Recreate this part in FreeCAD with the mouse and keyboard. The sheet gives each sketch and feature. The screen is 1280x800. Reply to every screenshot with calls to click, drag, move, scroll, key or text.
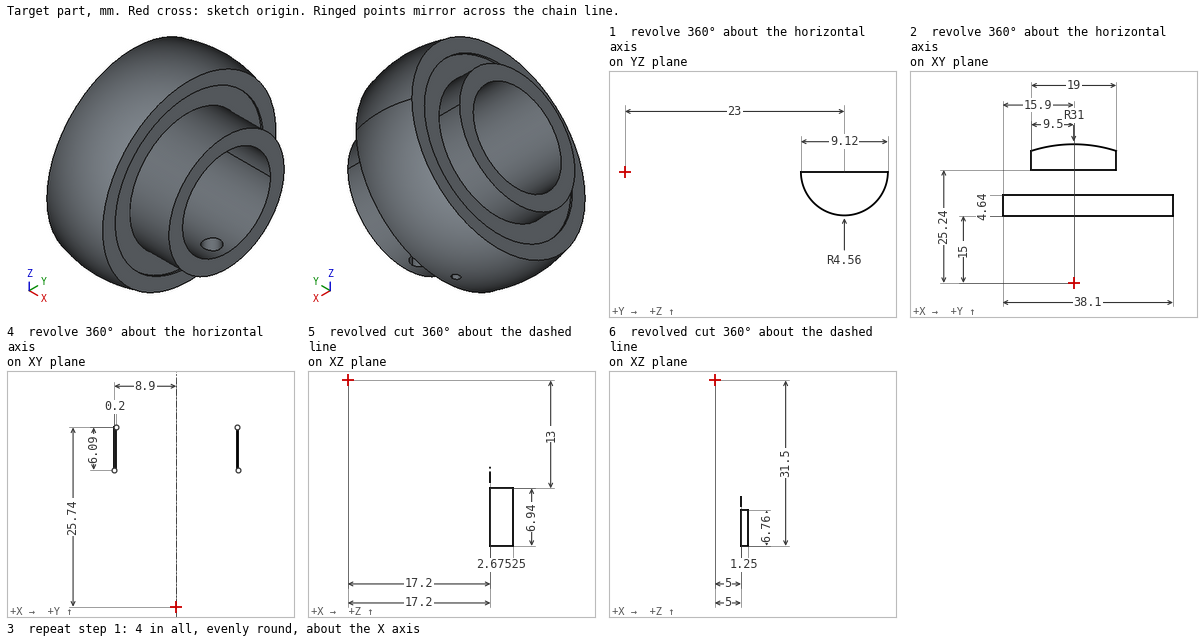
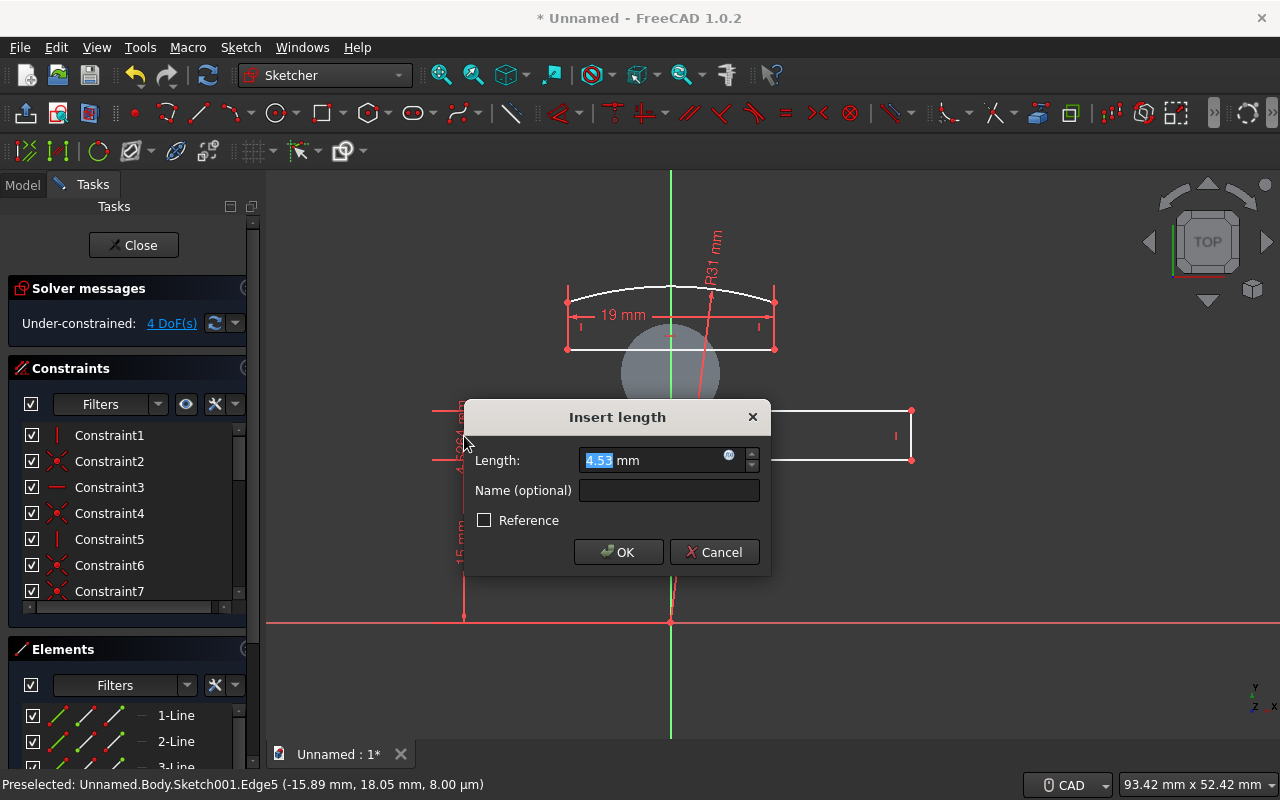
text(4.64)
key(Return)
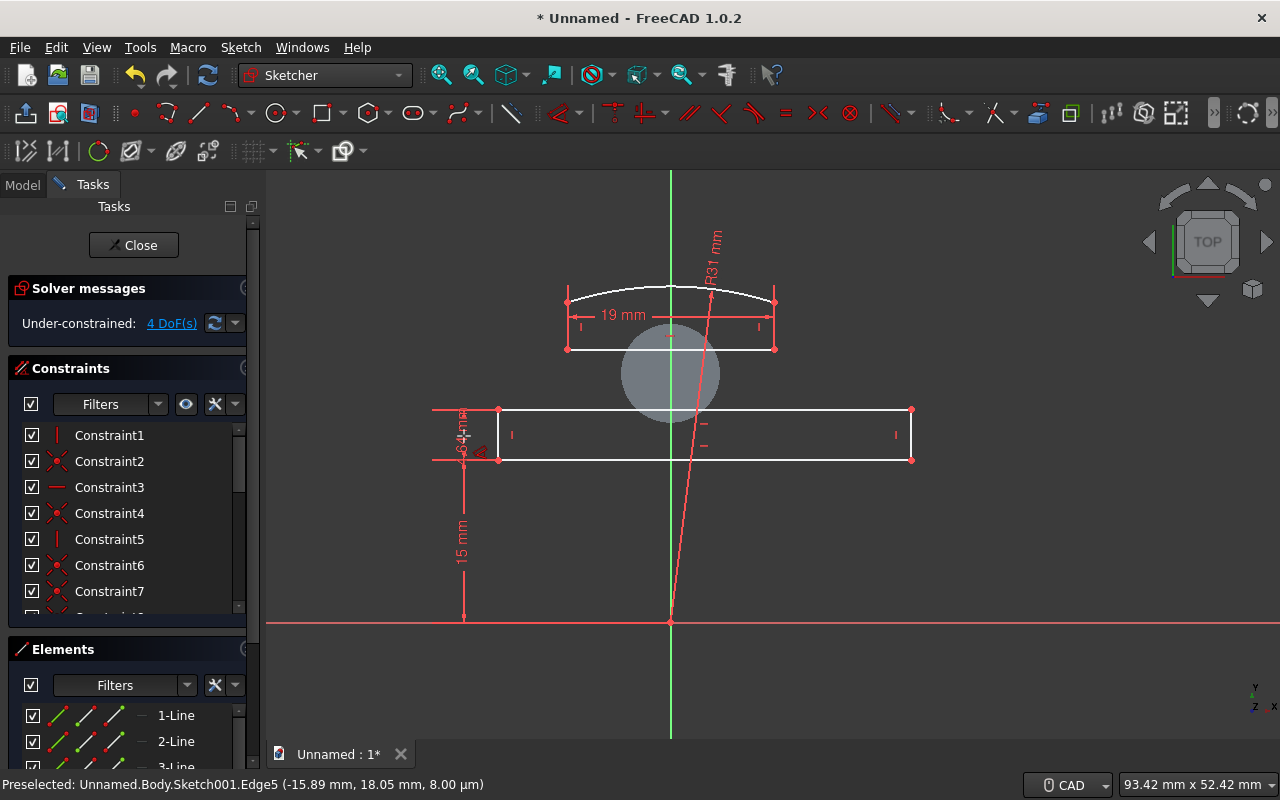
click(622, 460)
click(705, 494)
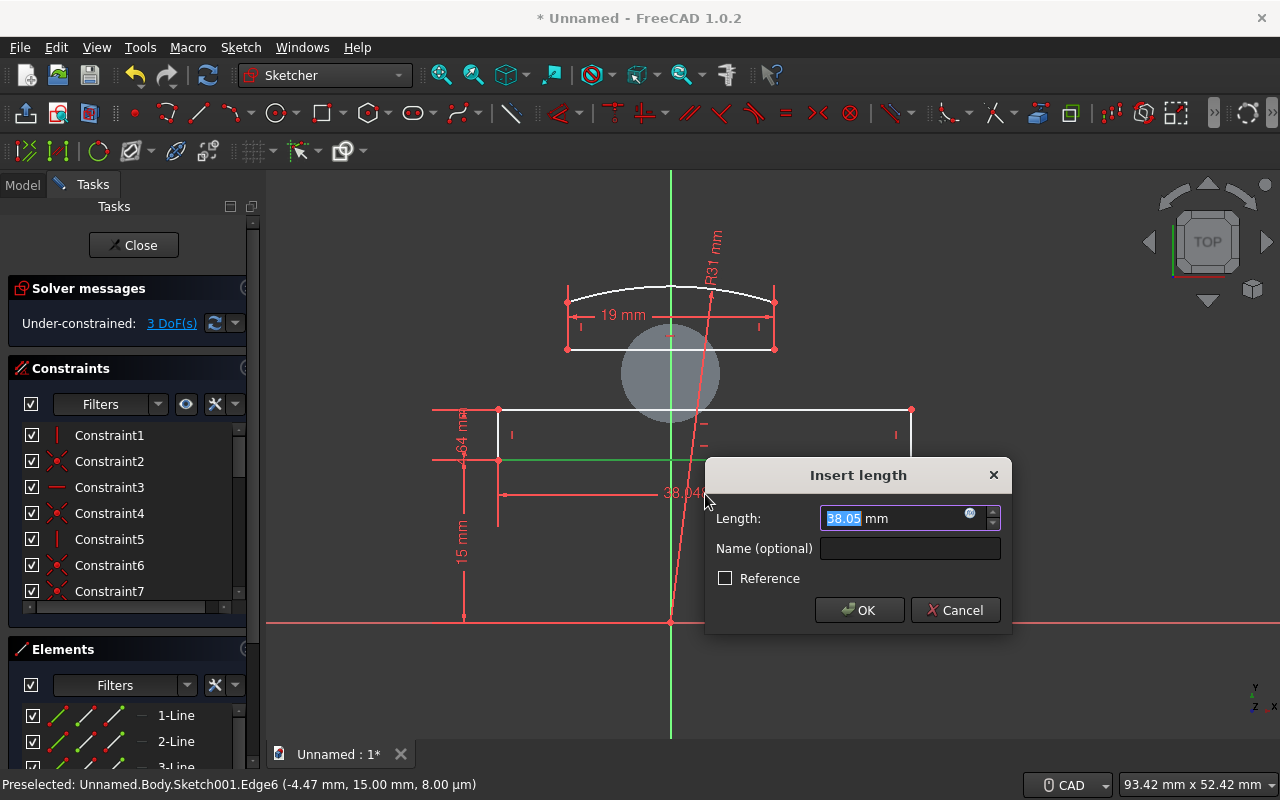
text(38.1)
key(Return)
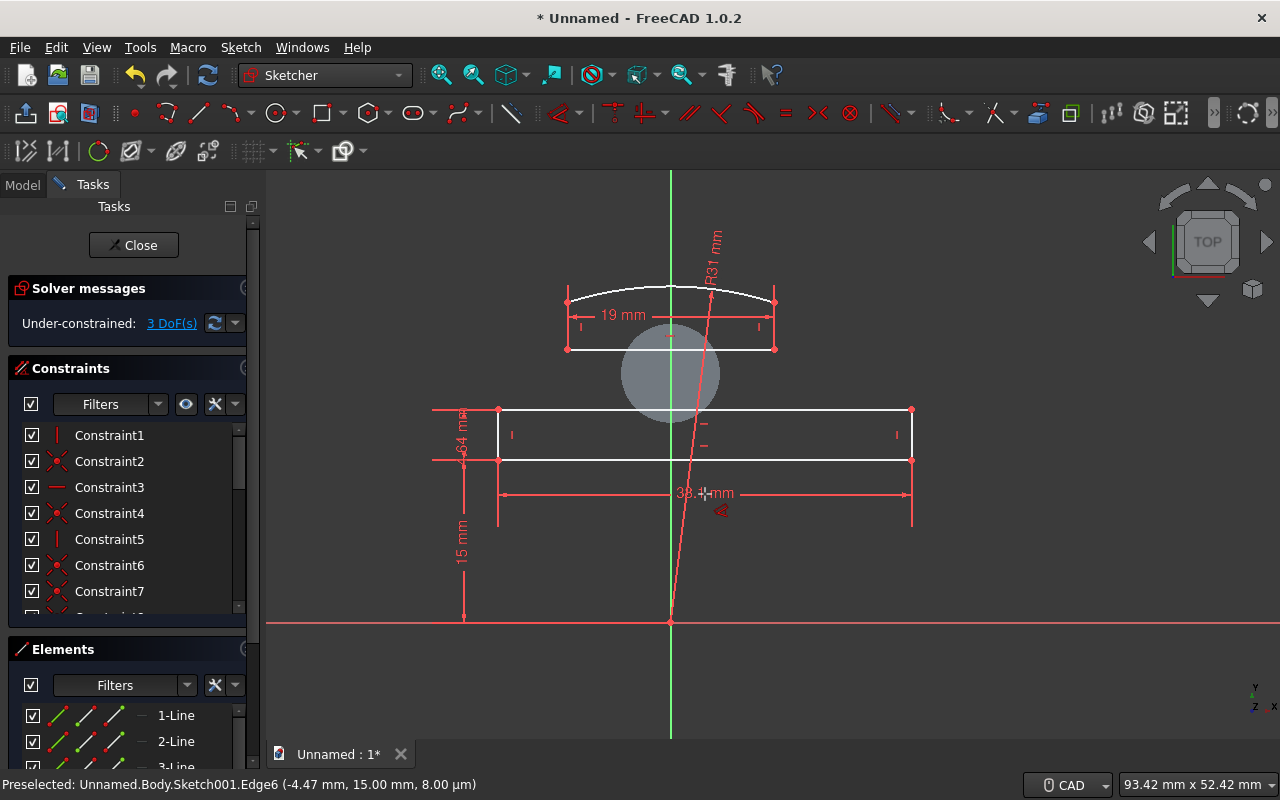
click(568, 303)
click(619, 657)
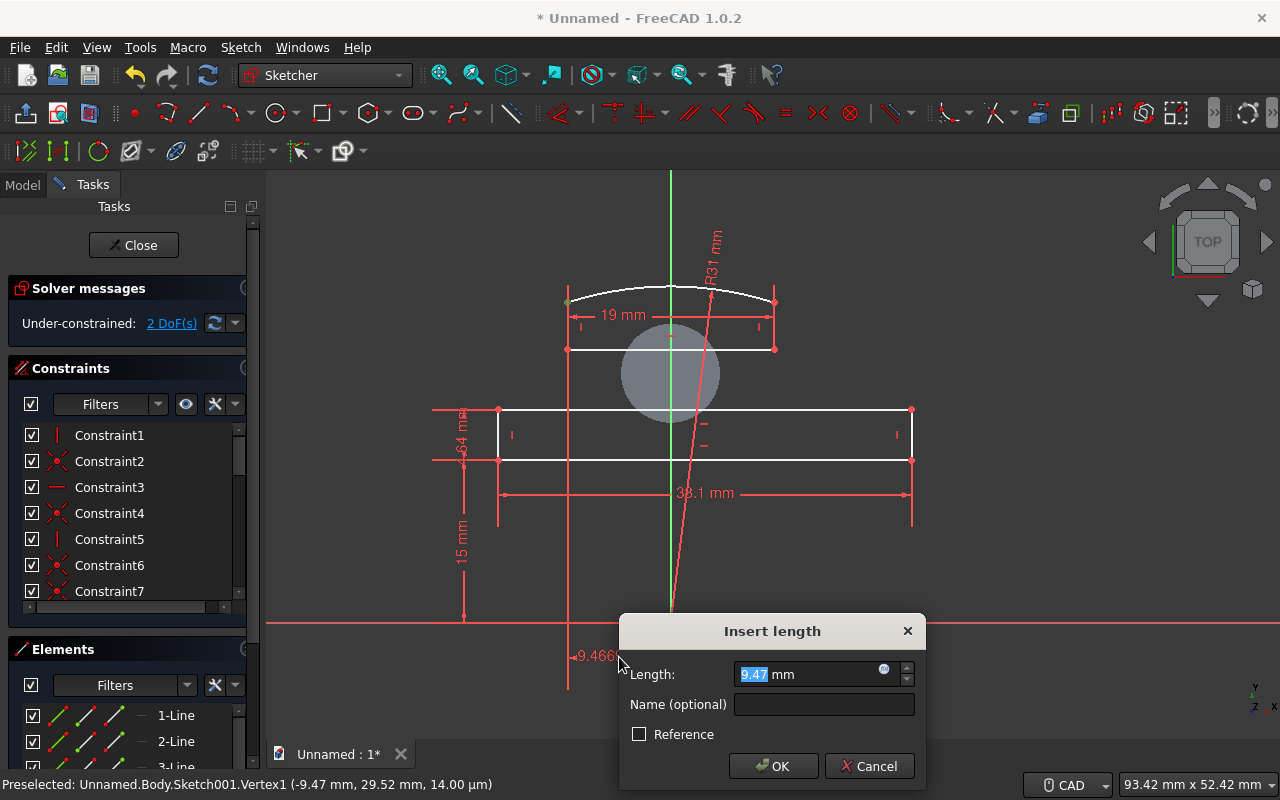
text(9.5)
key(Return)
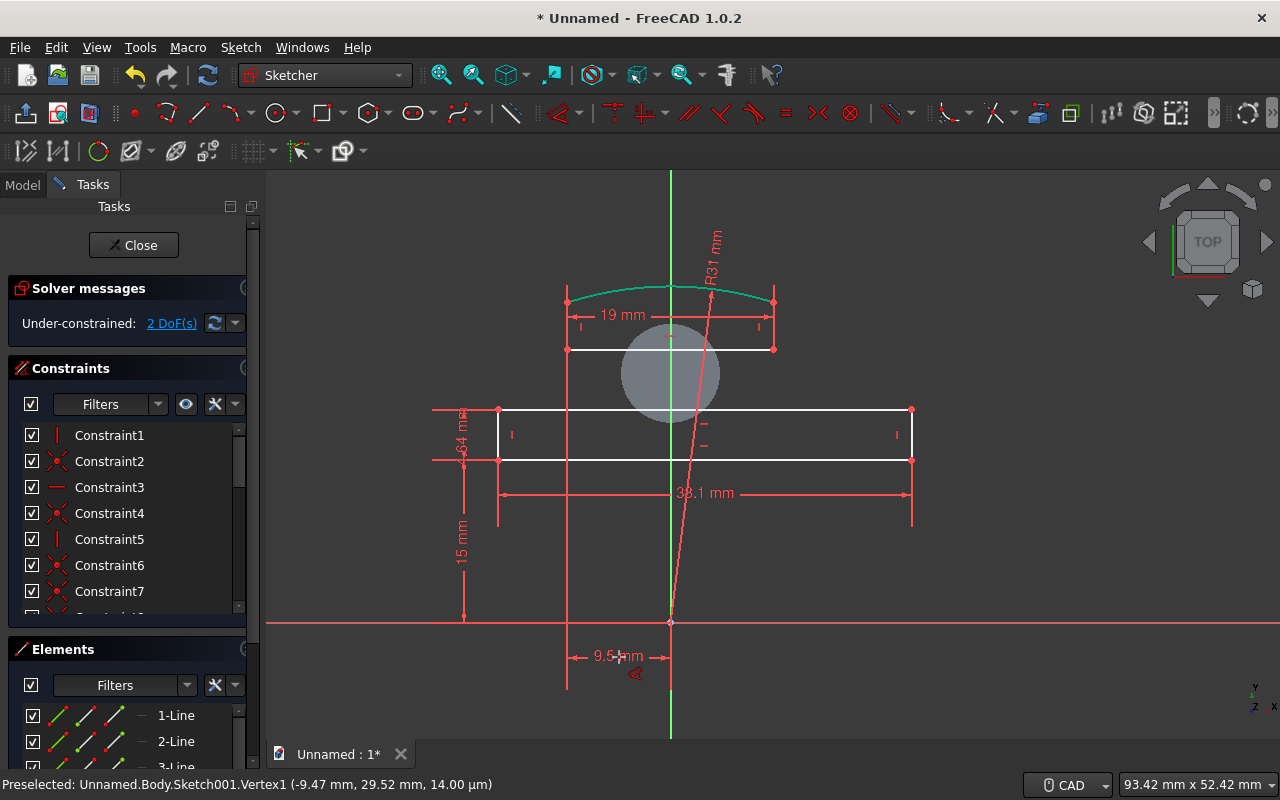
click(498, 410)
click(545, 657)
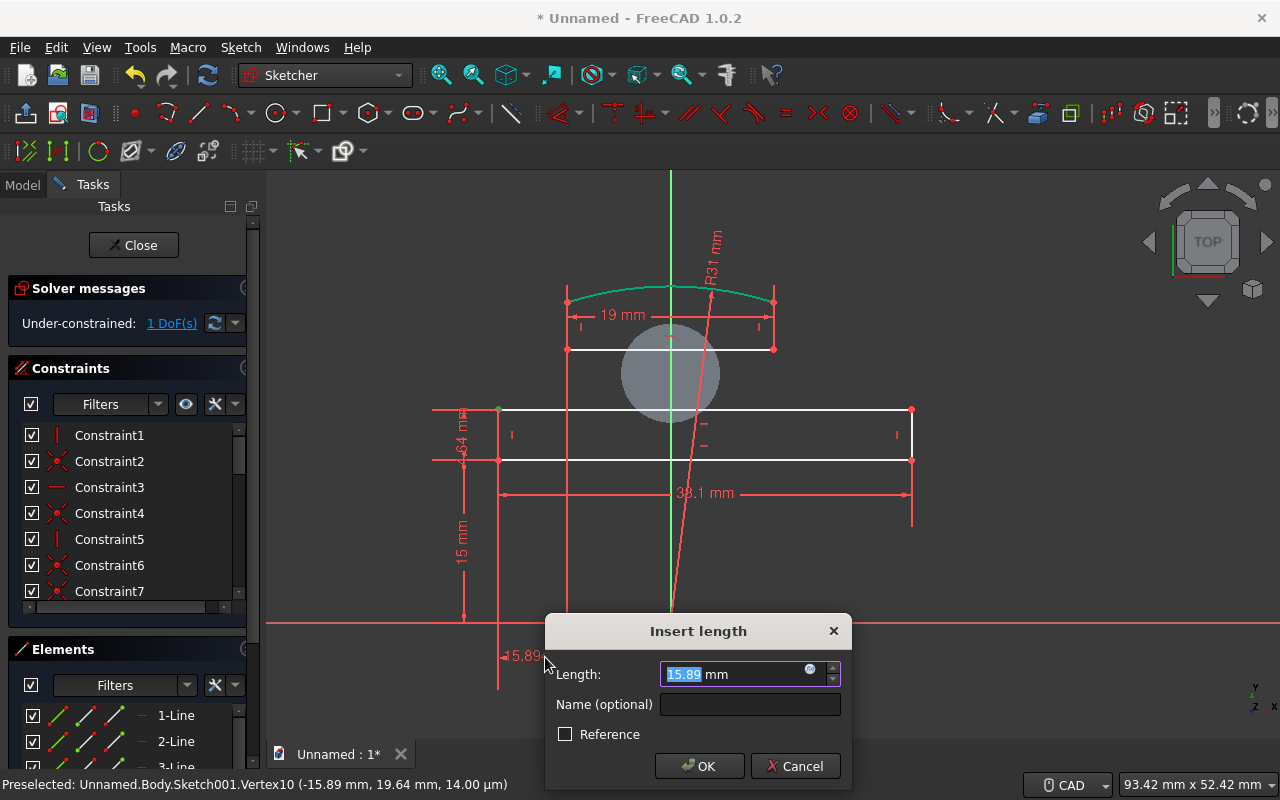
text(15.9)
key(Return)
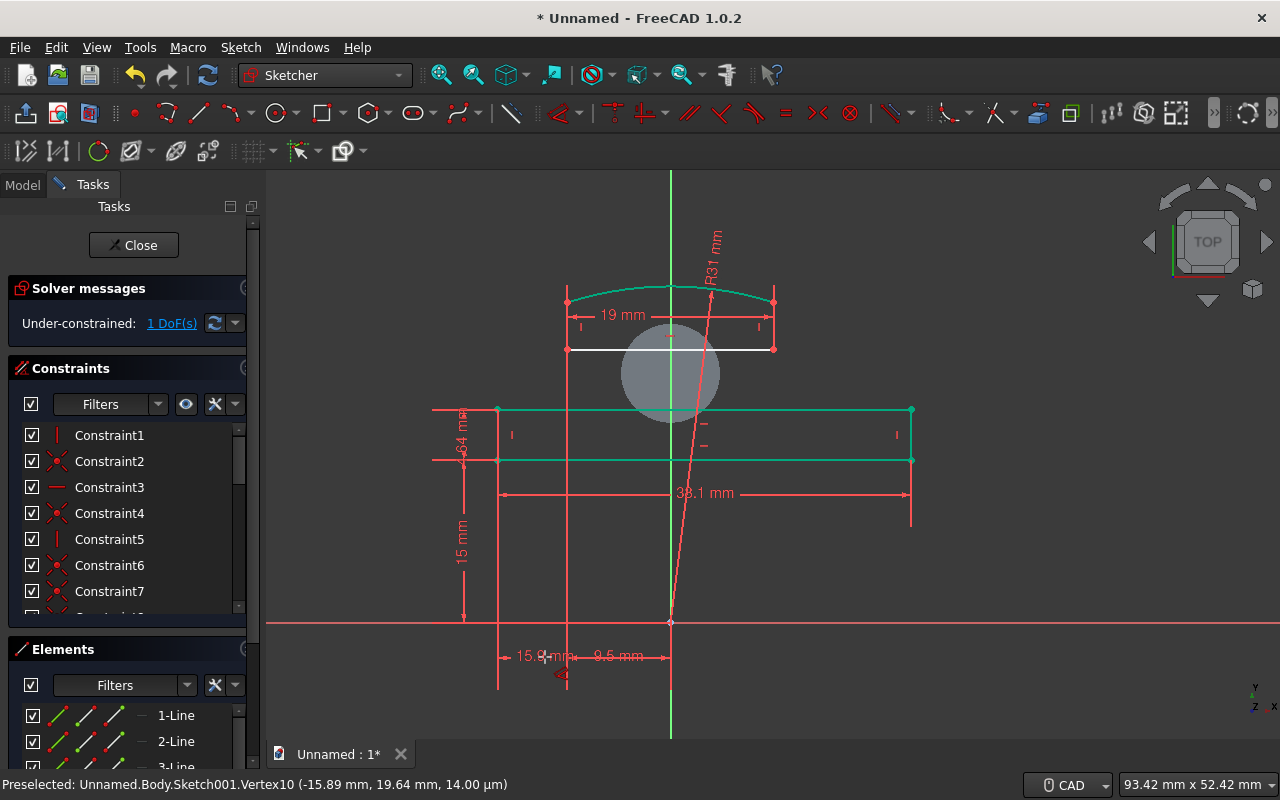
click(567, 350)
click(533, 486)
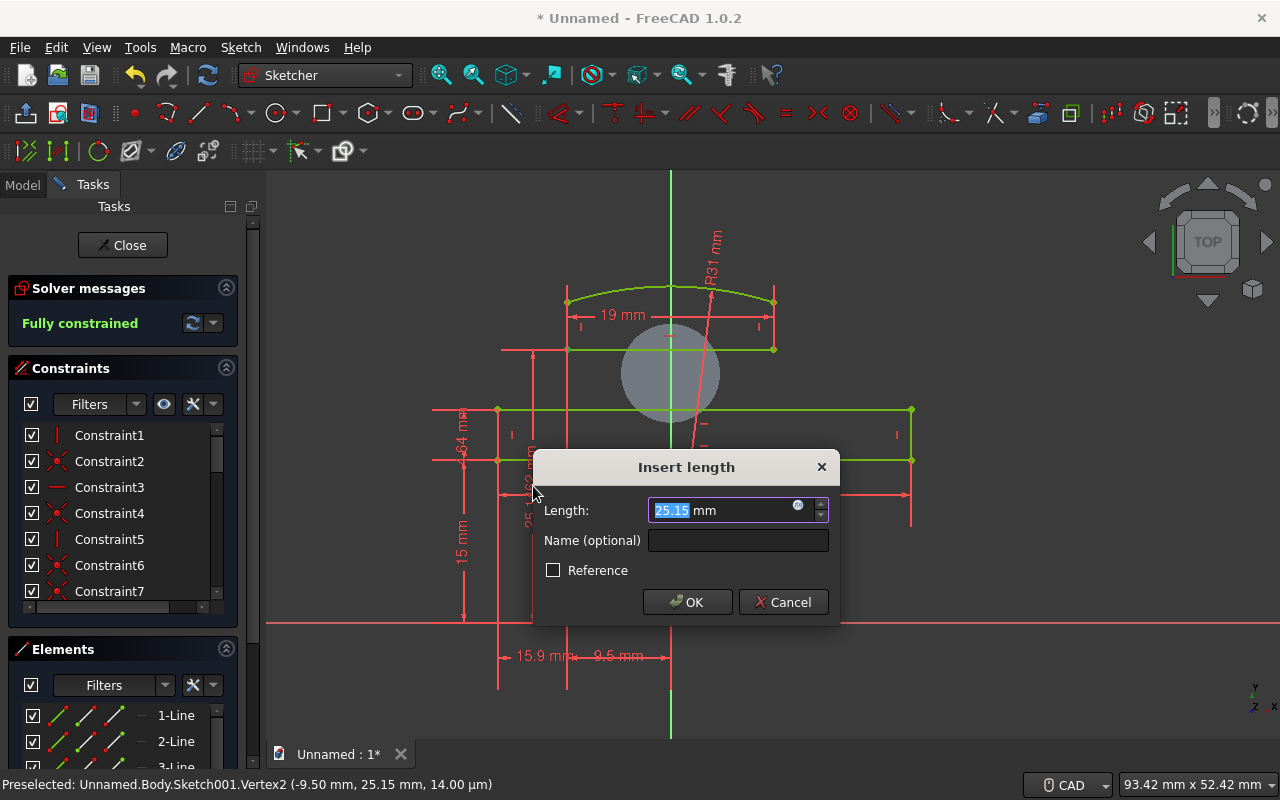
text(25.24)
key(Return)
key(Escape)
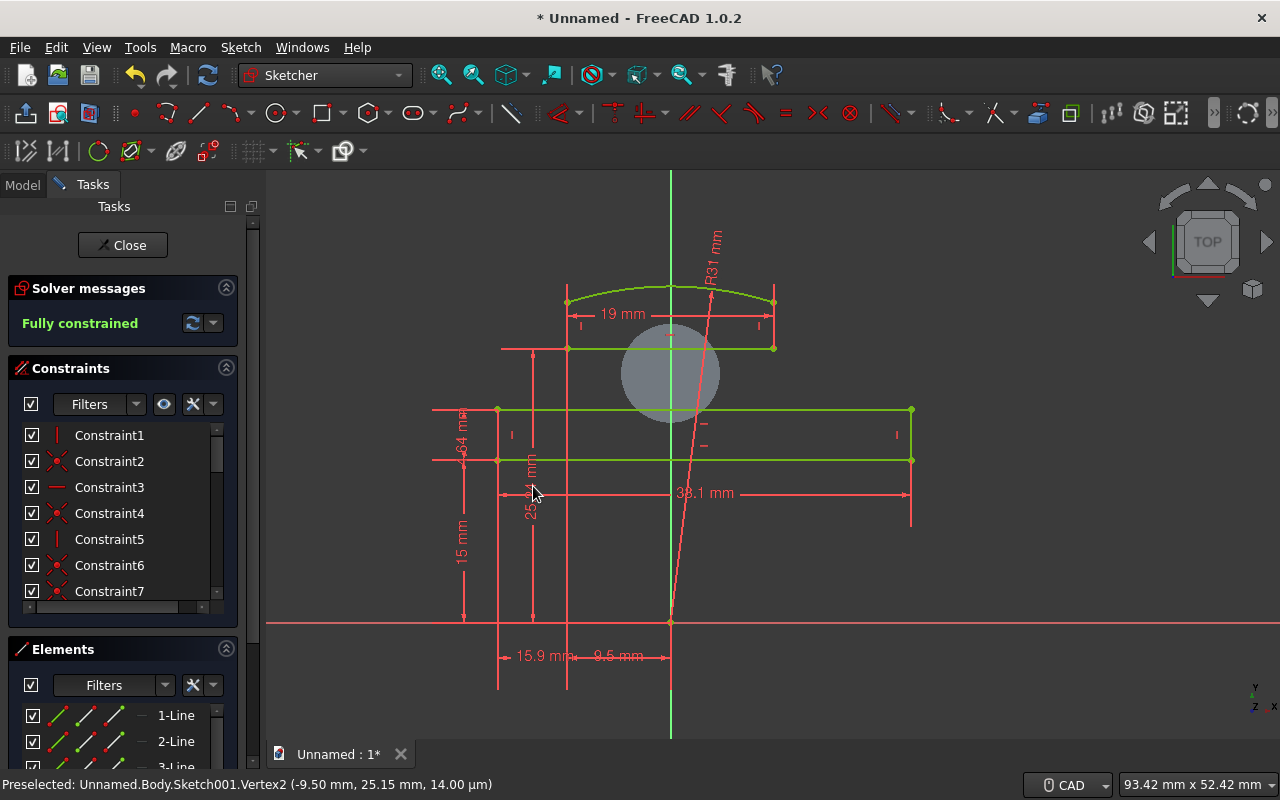
click(123, 245)